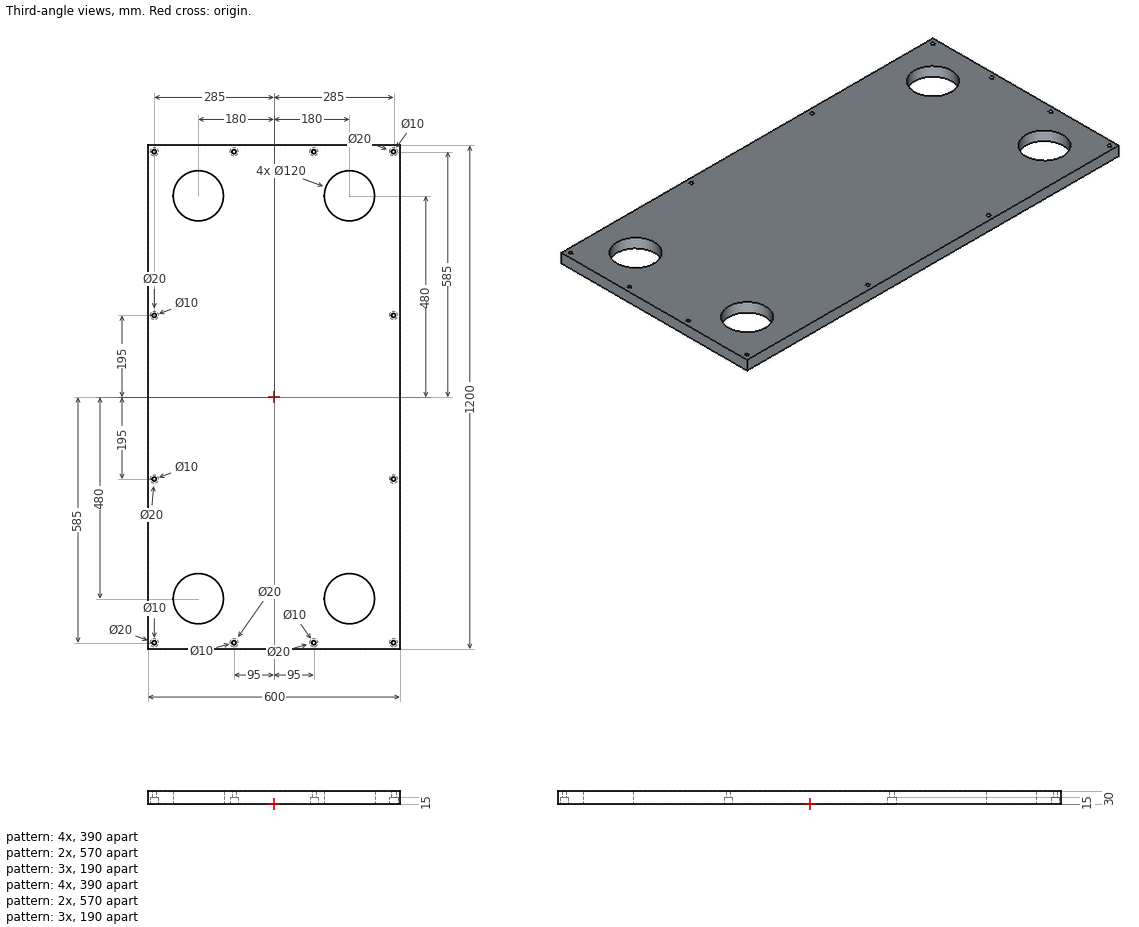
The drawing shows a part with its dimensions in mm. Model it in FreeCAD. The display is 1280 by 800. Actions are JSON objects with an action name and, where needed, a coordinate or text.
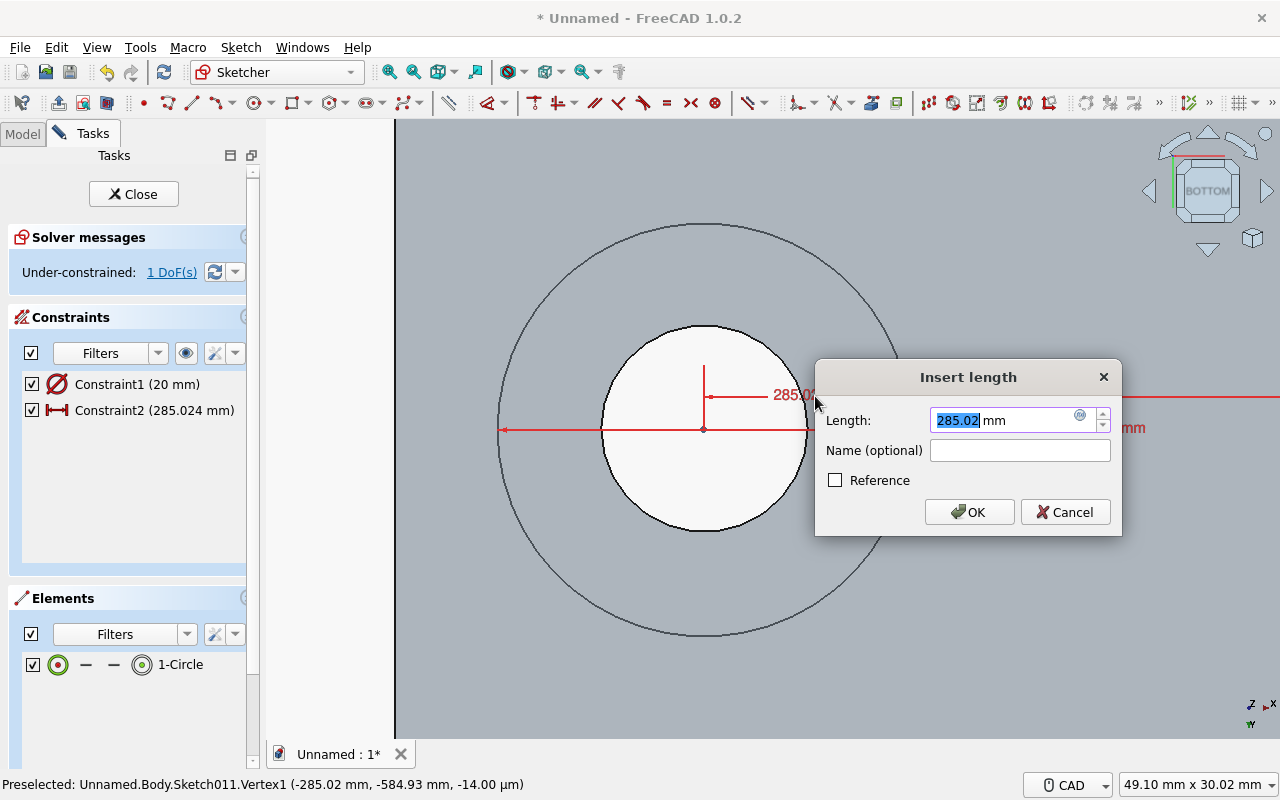
{"action": "type", "text": "285"}
{"action": "key", "text": "Return"}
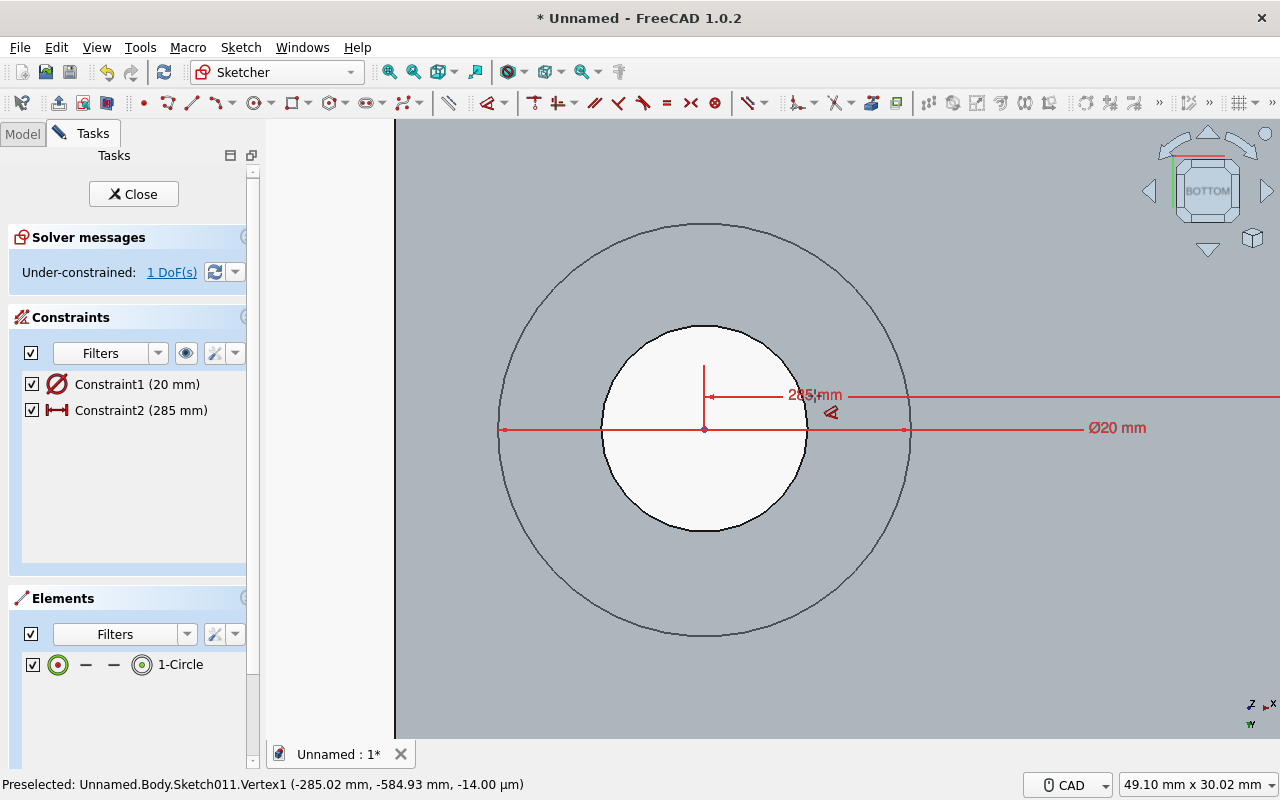
{"action": "left_click", "coordinate": [704, 430]}
{"action": "left_click", "coordinate": [670, 570]}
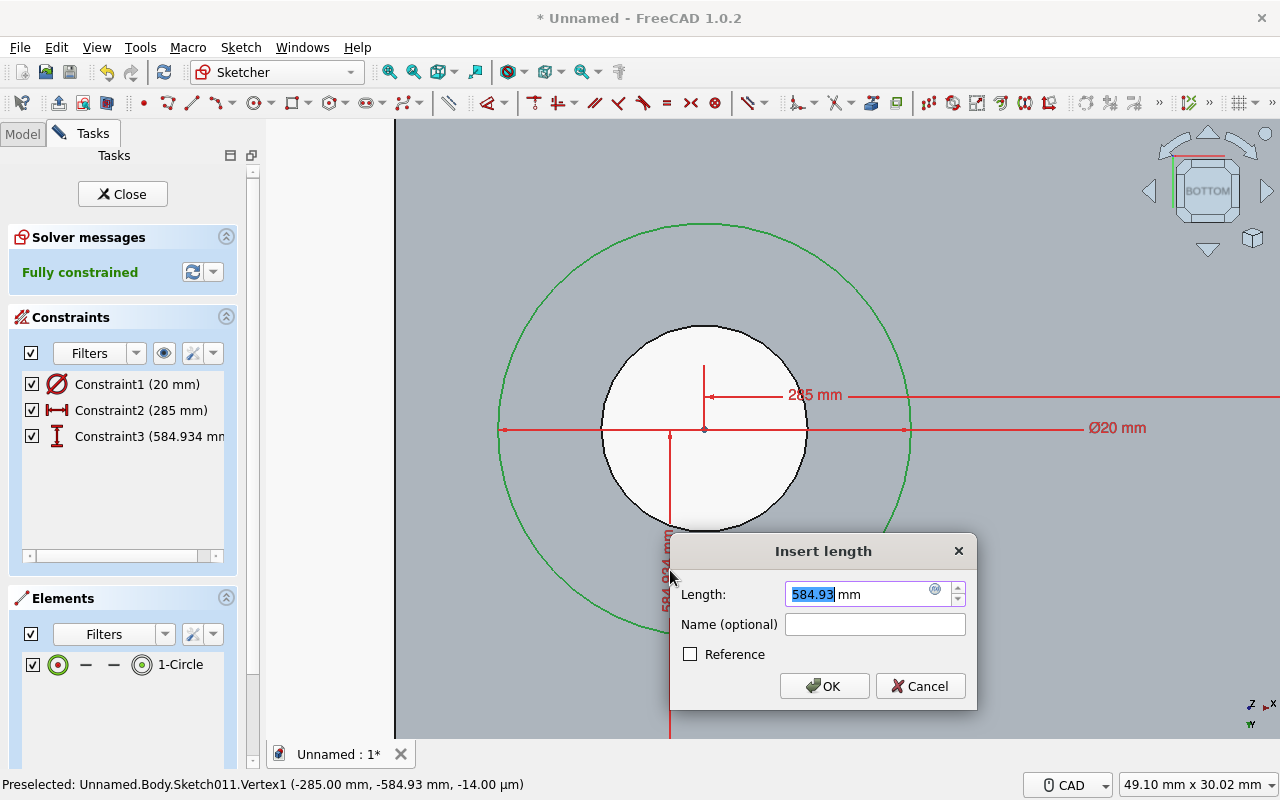
{"action": "type", "text": "585"}
{"action": "key", "text": "Return"}
{"action": "key", "text": "Escape"}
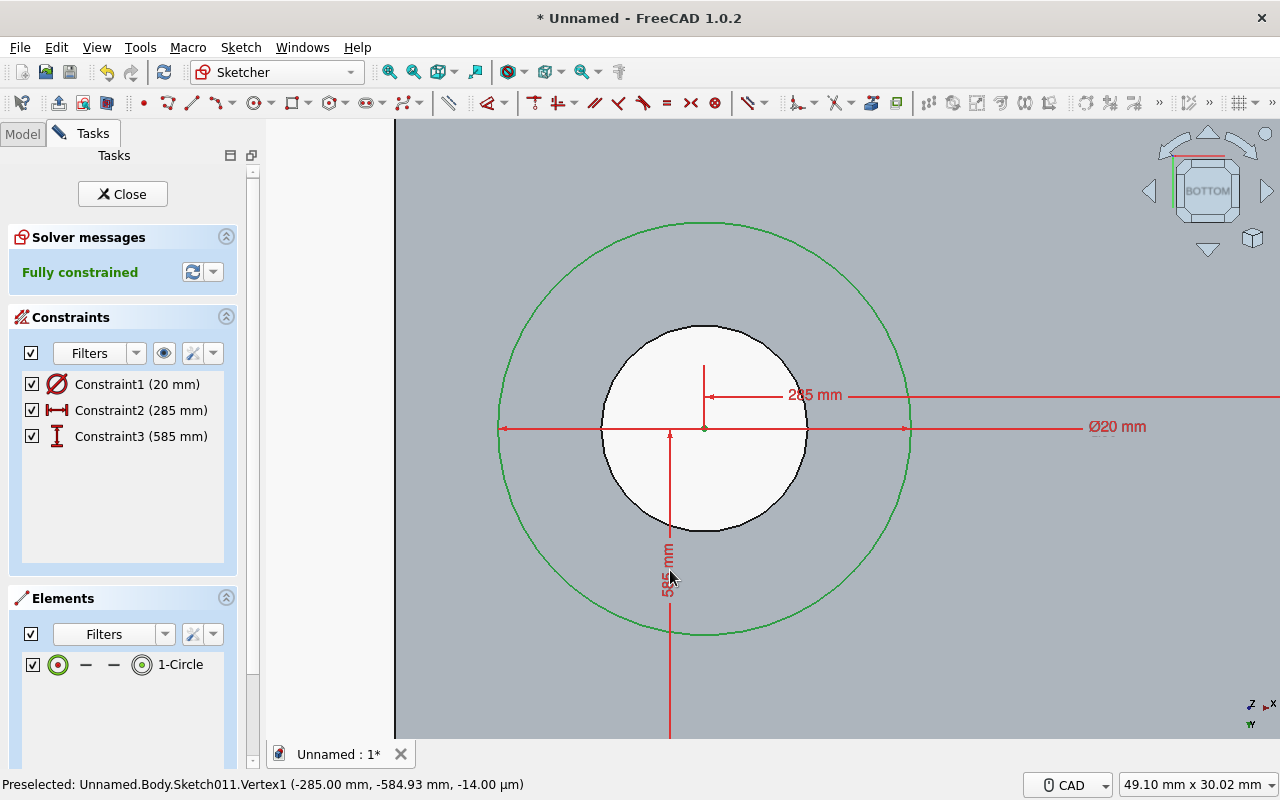
{"action": "left_click", "coordinate": [123, 194]}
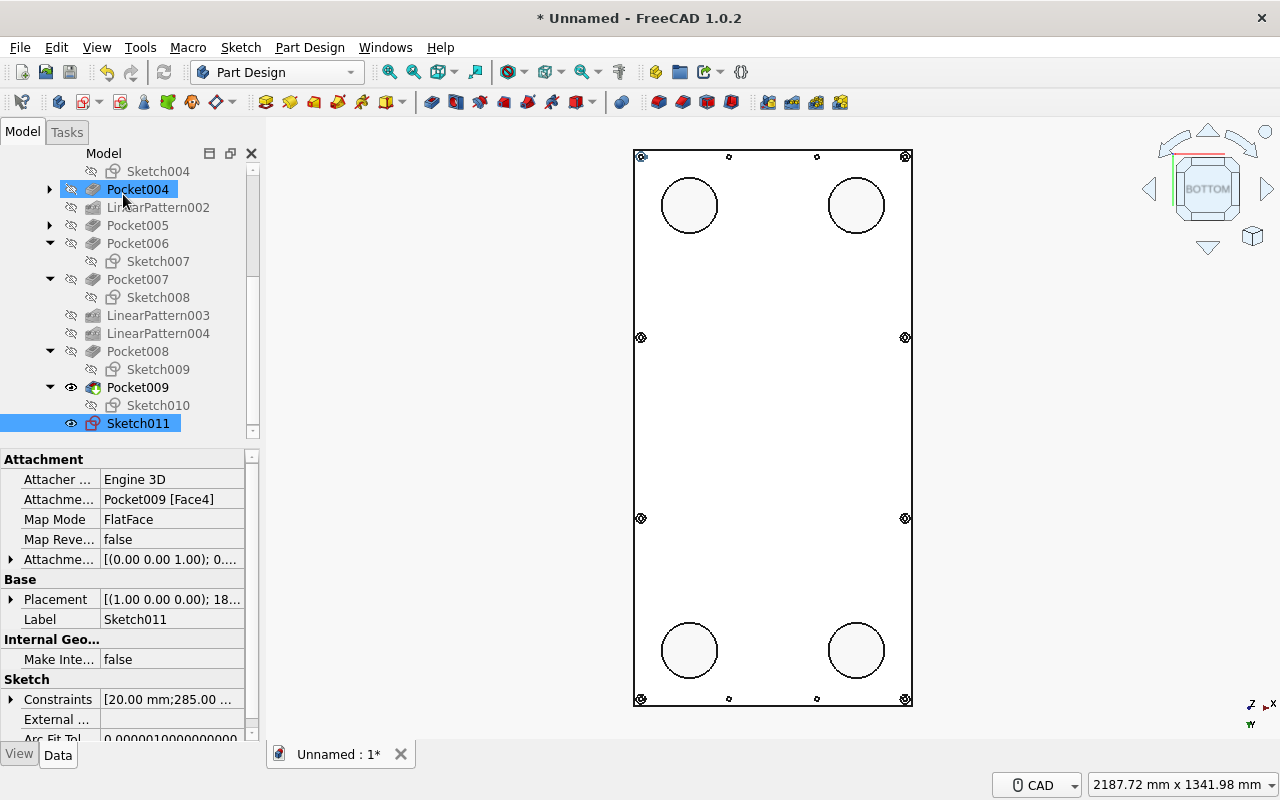
{"action": "left_click", "coordinate": [432, 102]}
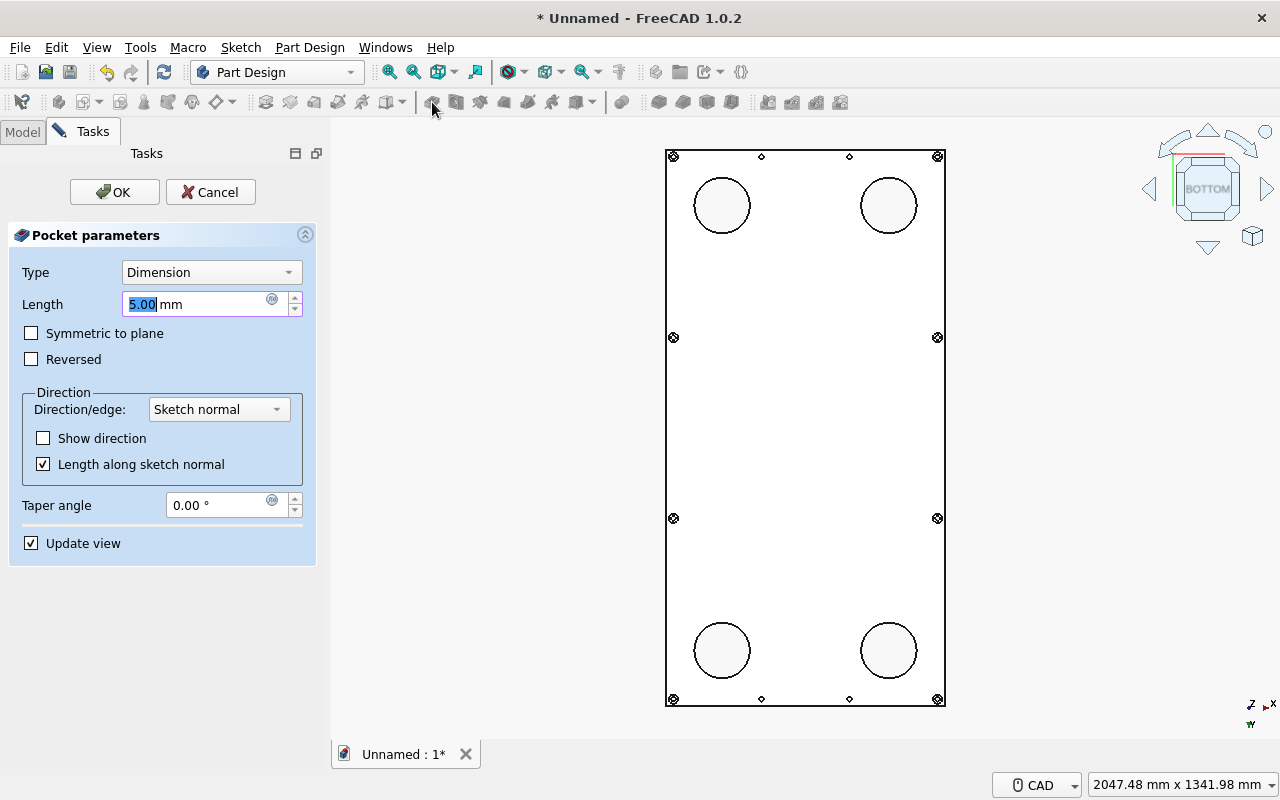
{"action": "type", "text": "15"}
{"action": "key", "text": "Tab"}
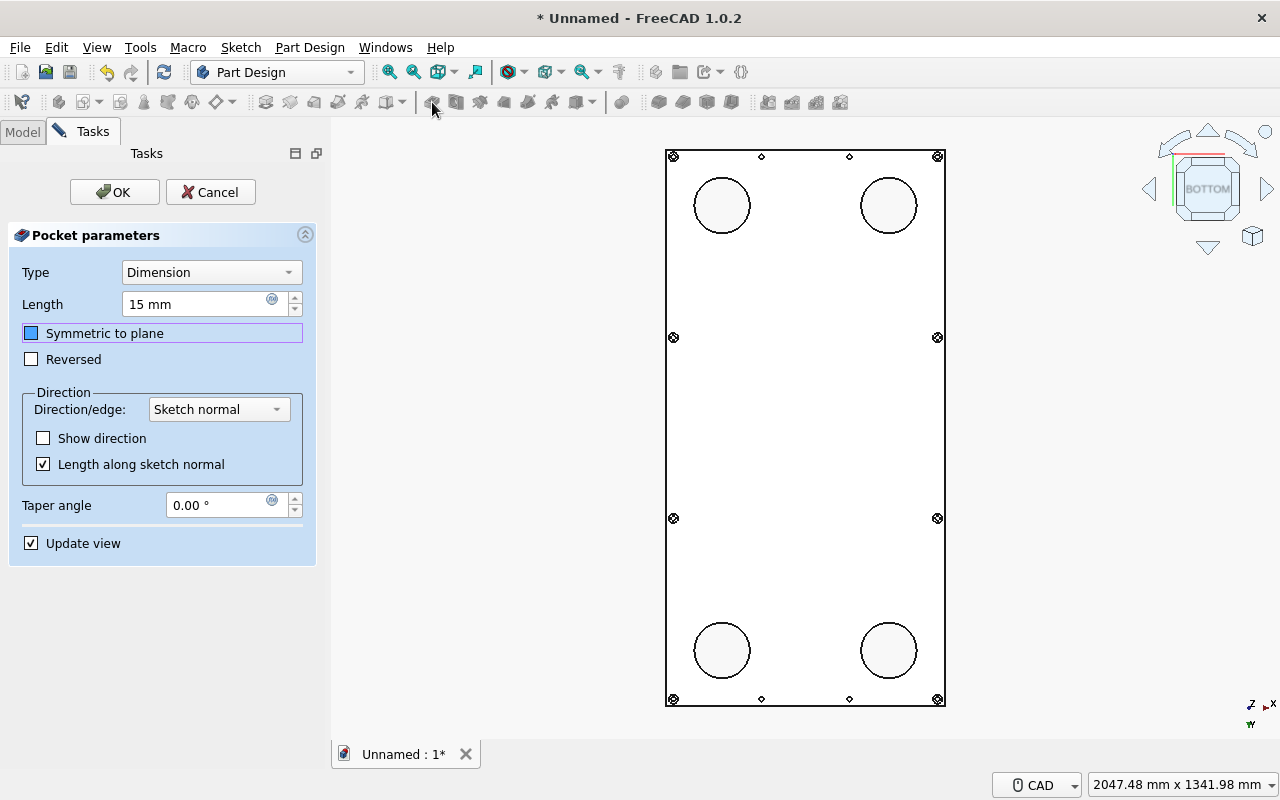
{"action": "left_click", "coordinate": [115, 192]}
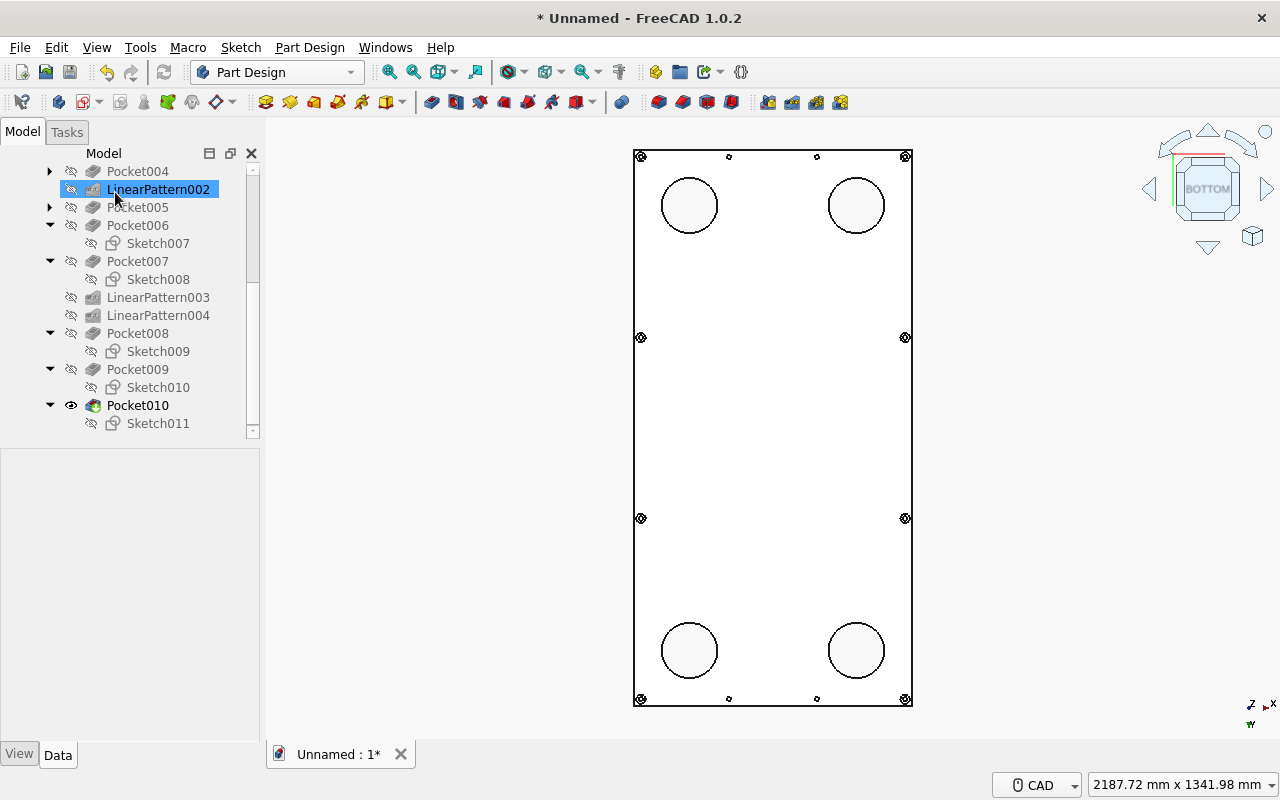
{"action": "left_click", "coordinate": [116, 261]}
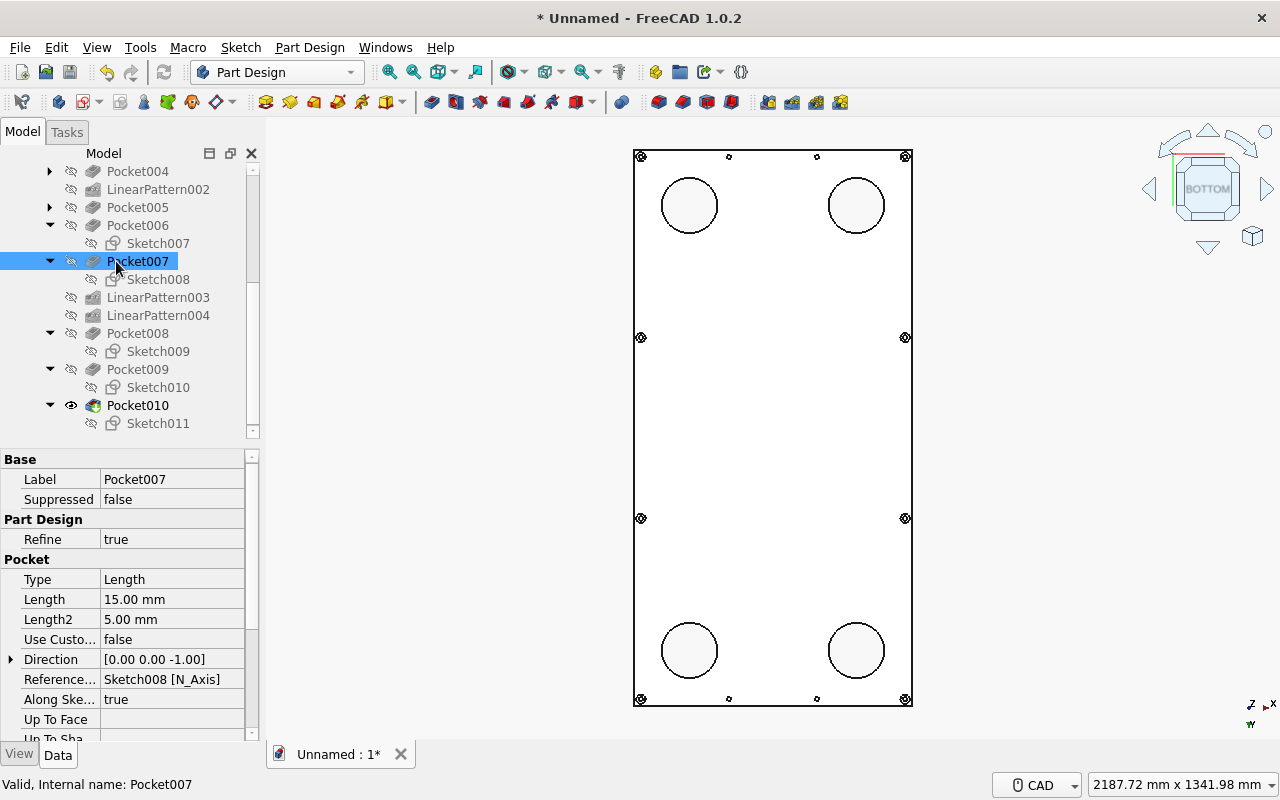
{"action": "left_click", "coordinate": [792, 102]}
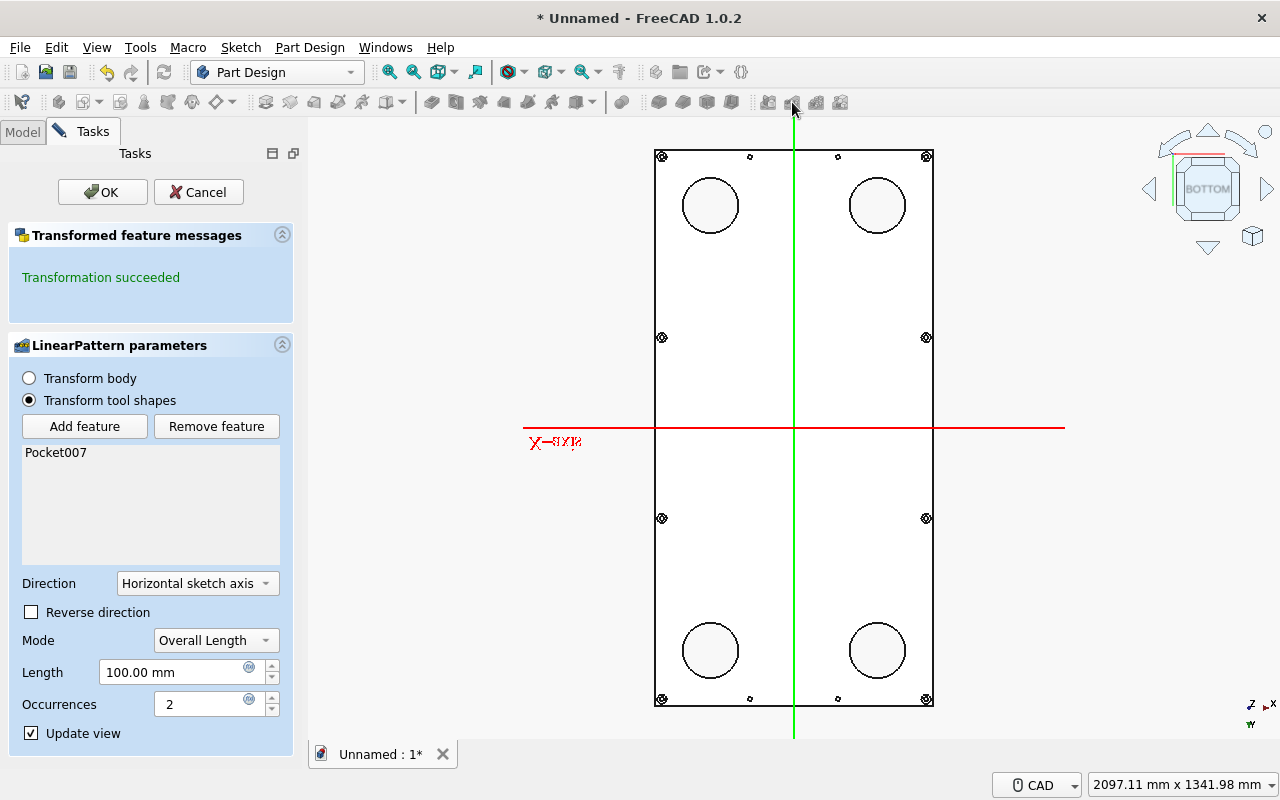
{"action": "left_click", "coordinate": [198, 584]}